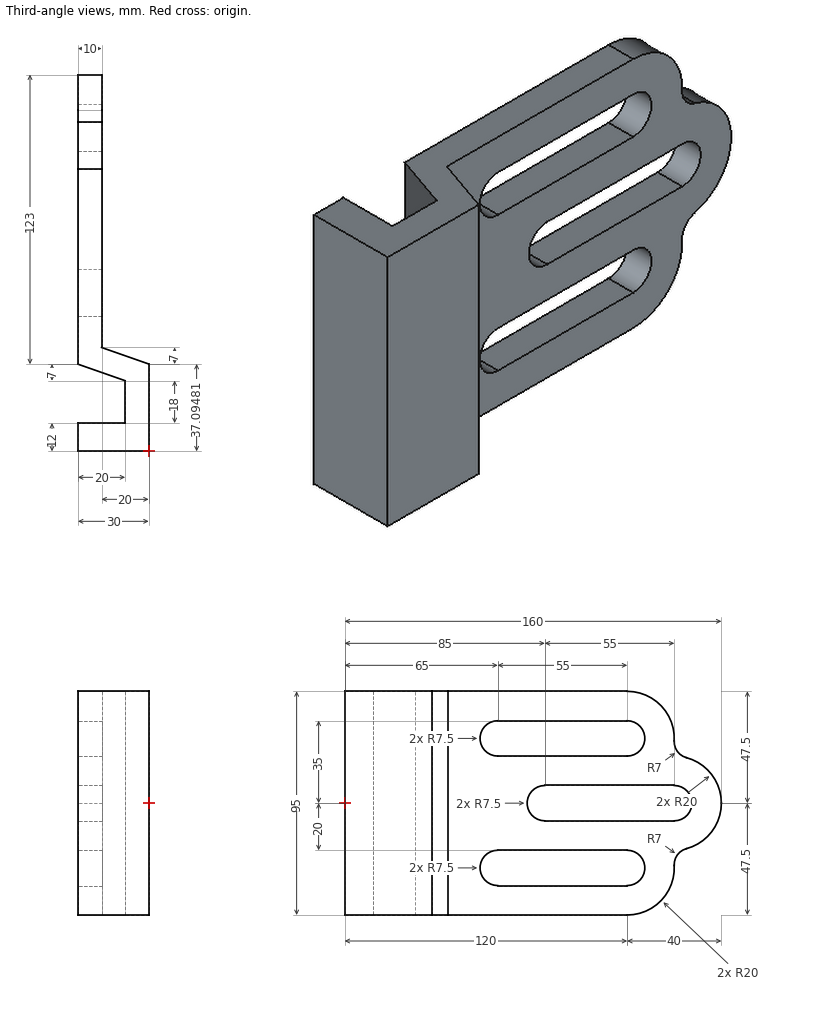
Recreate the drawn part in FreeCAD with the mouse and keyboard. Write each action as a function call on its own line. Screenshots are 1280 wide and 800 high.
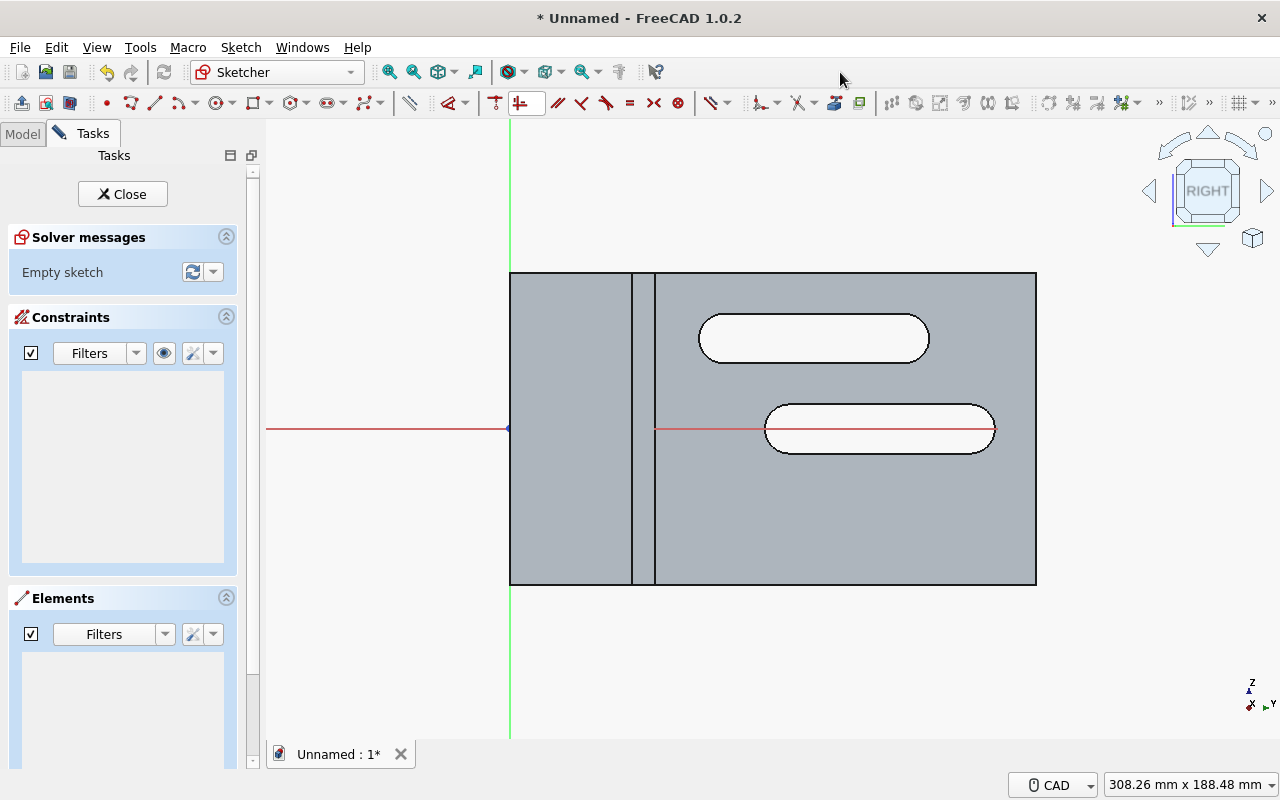
scroll(750, 604, up, 2)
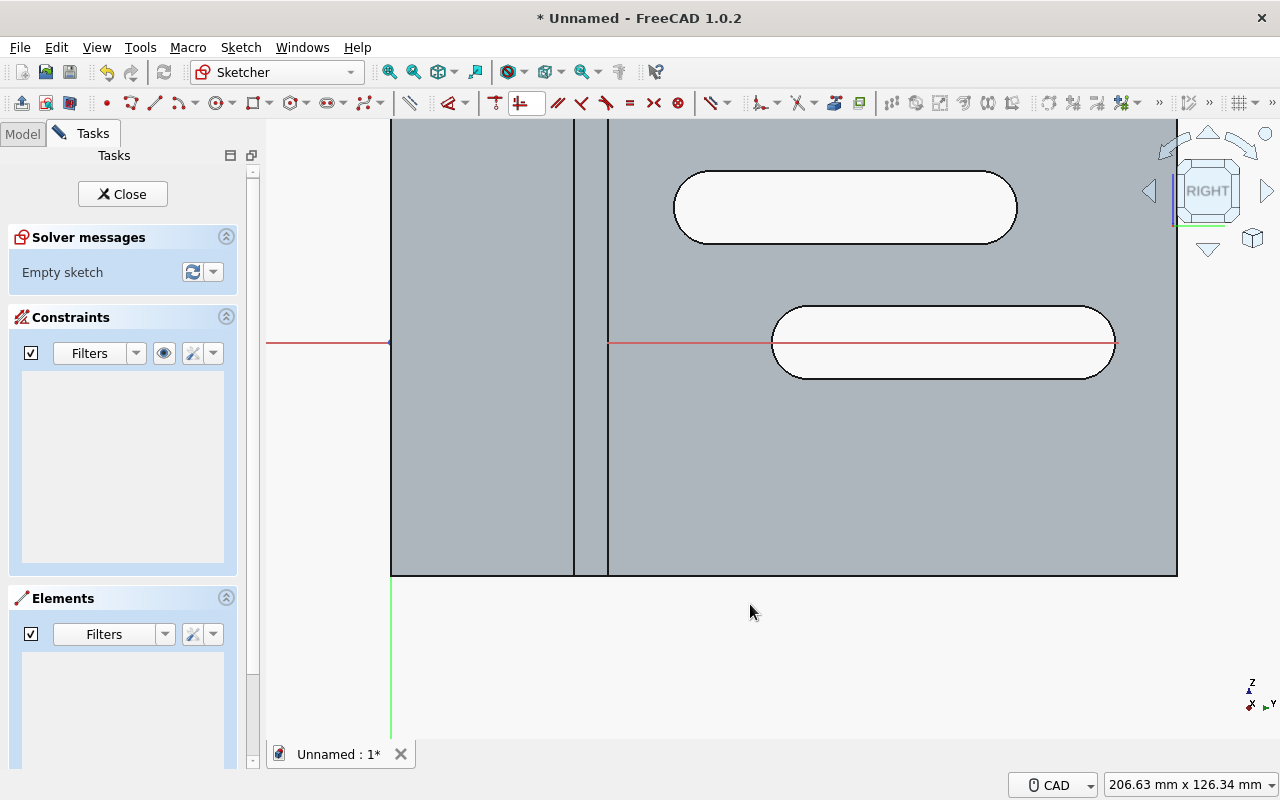
key(g)
key(s)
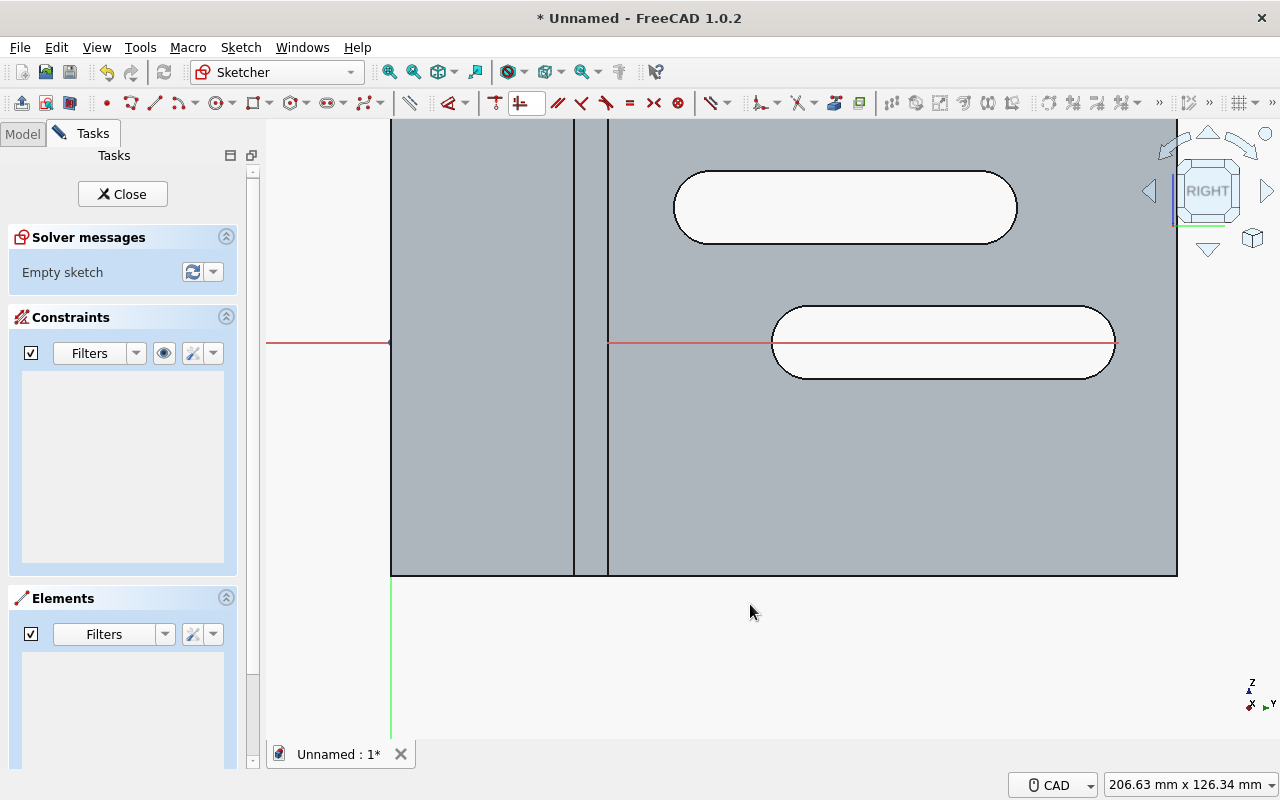
click(710, 477)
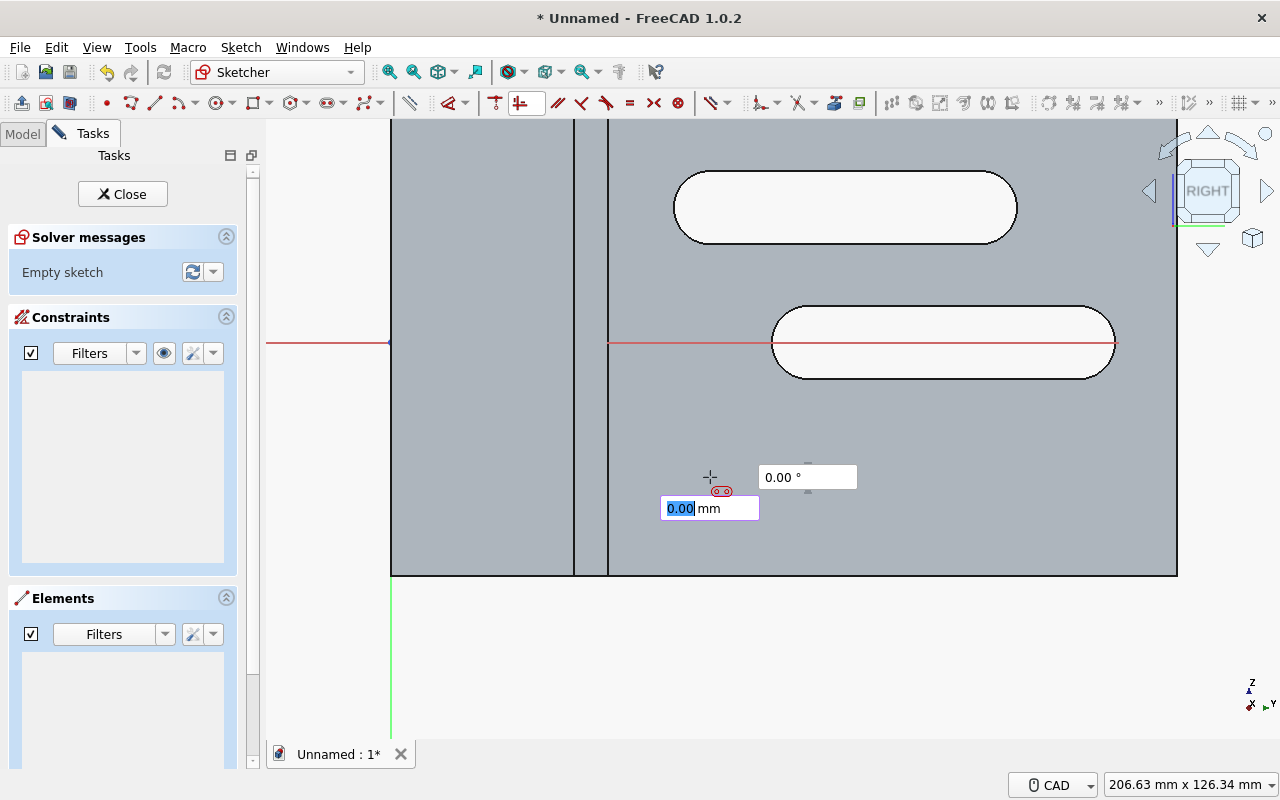
click(980, 477)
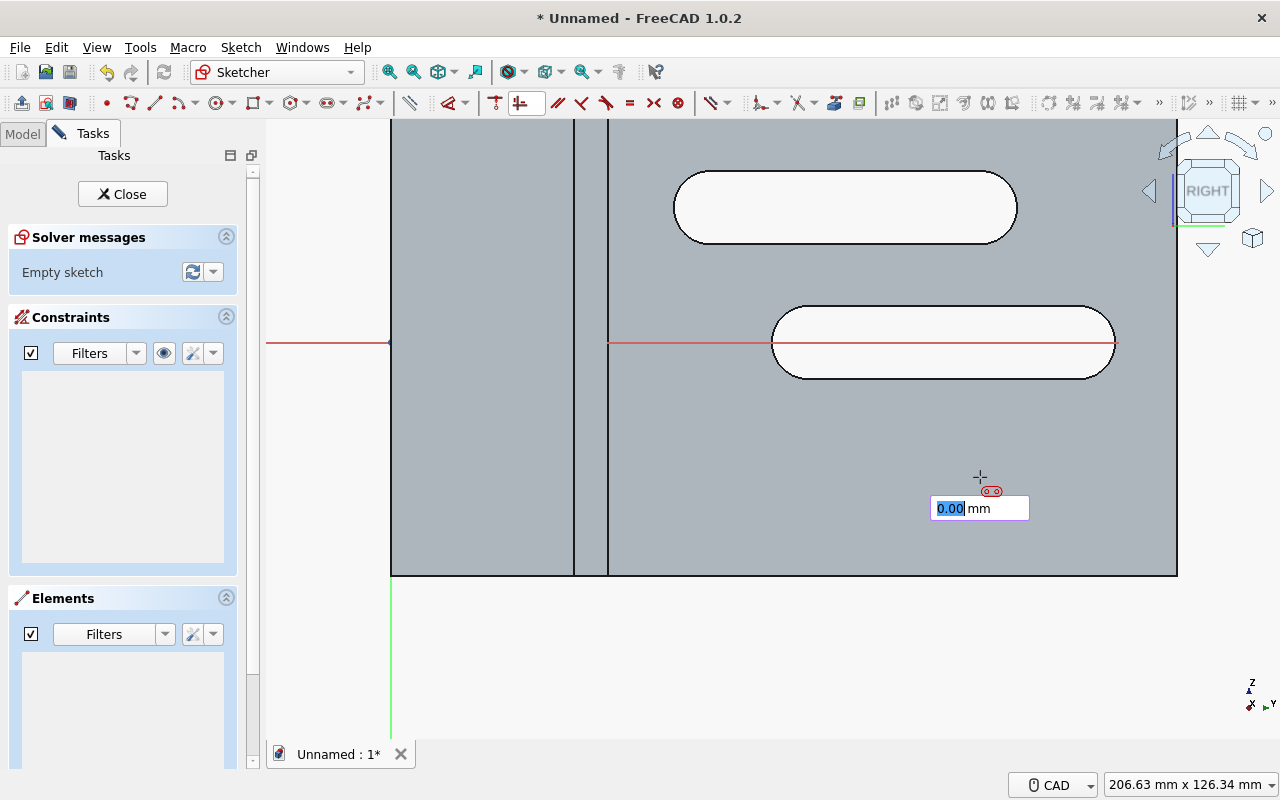
click(845, 514)
key(Escape)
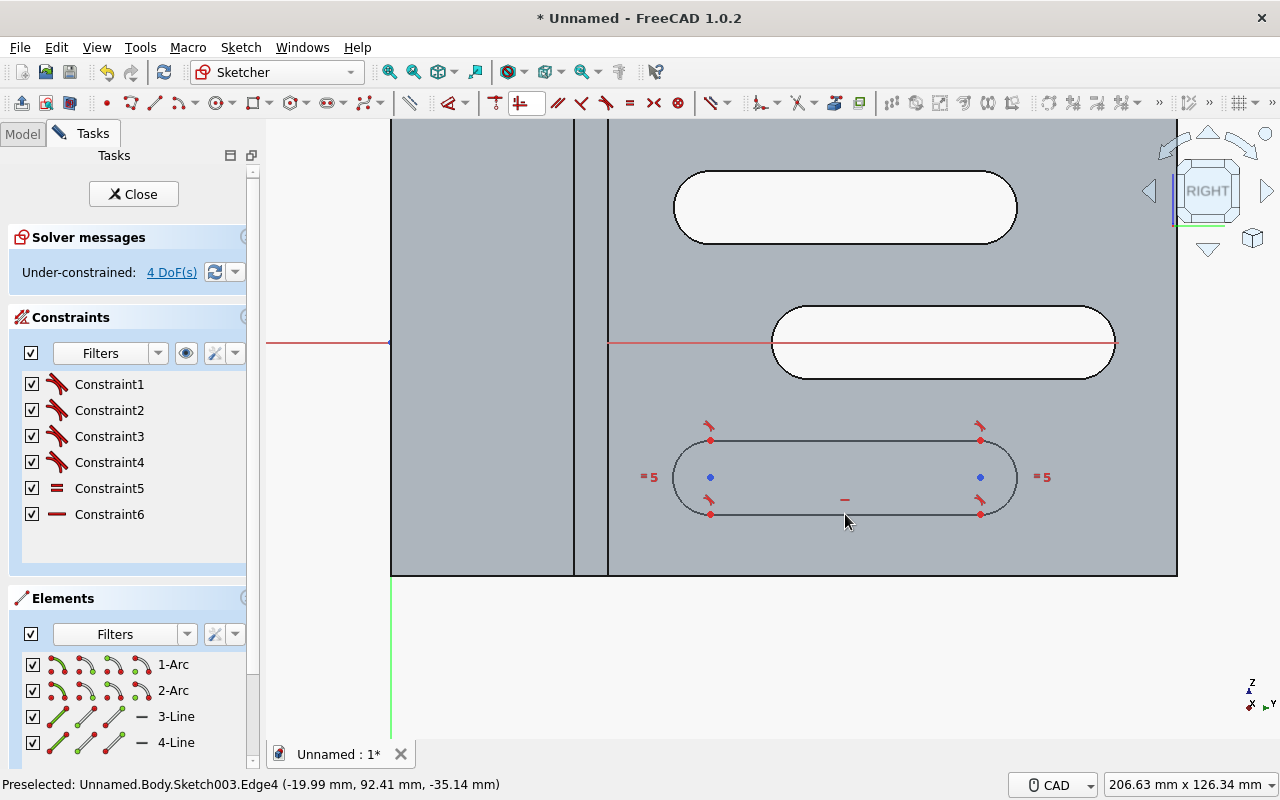
click(448, 104)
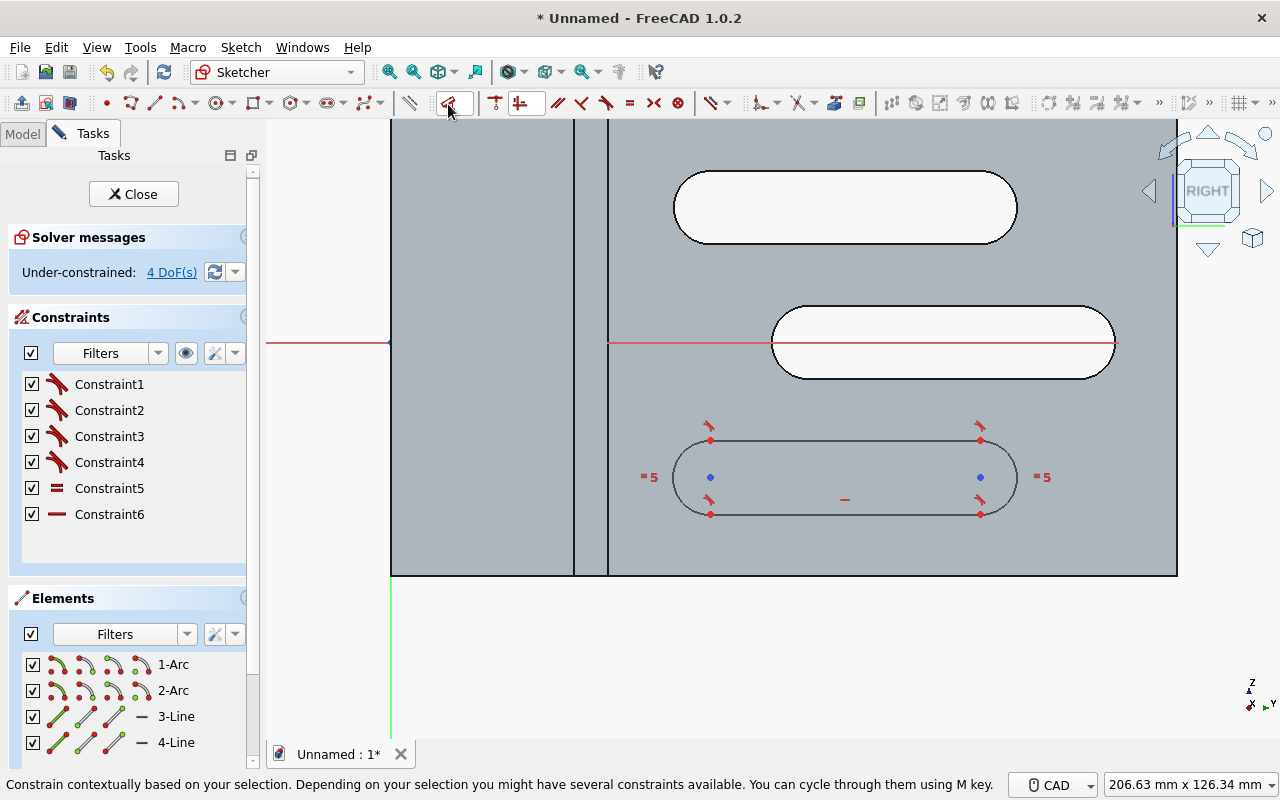
click(680, 456)
click(654, 437)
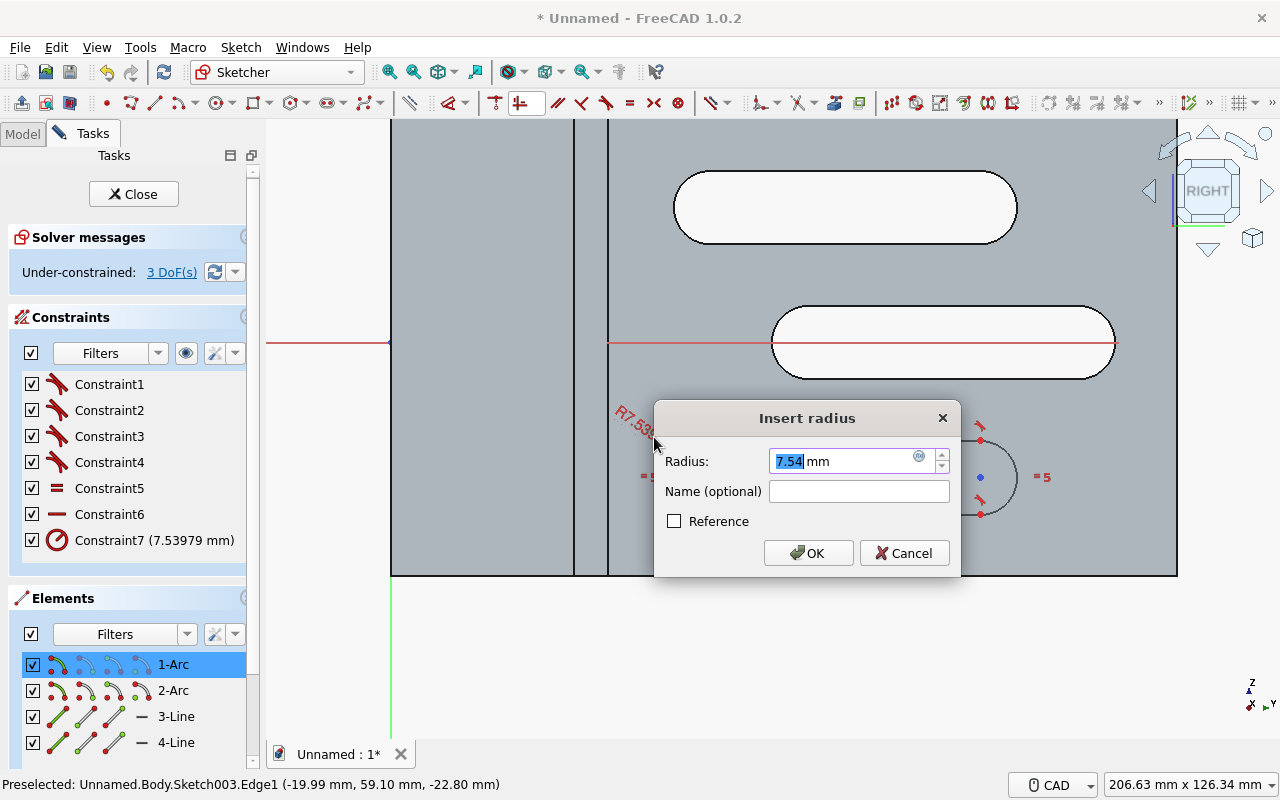
text(7.5)
key(Return)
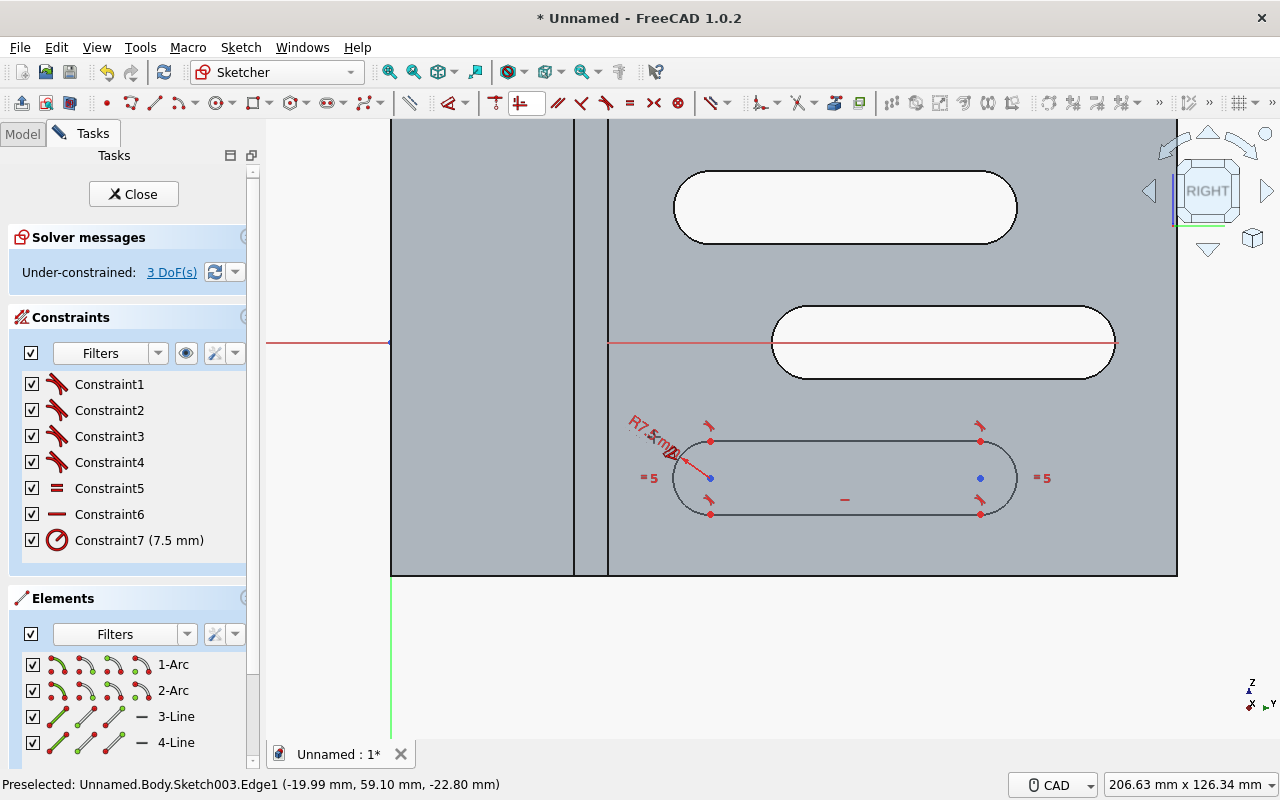
click(791, 441)
click(845, 475)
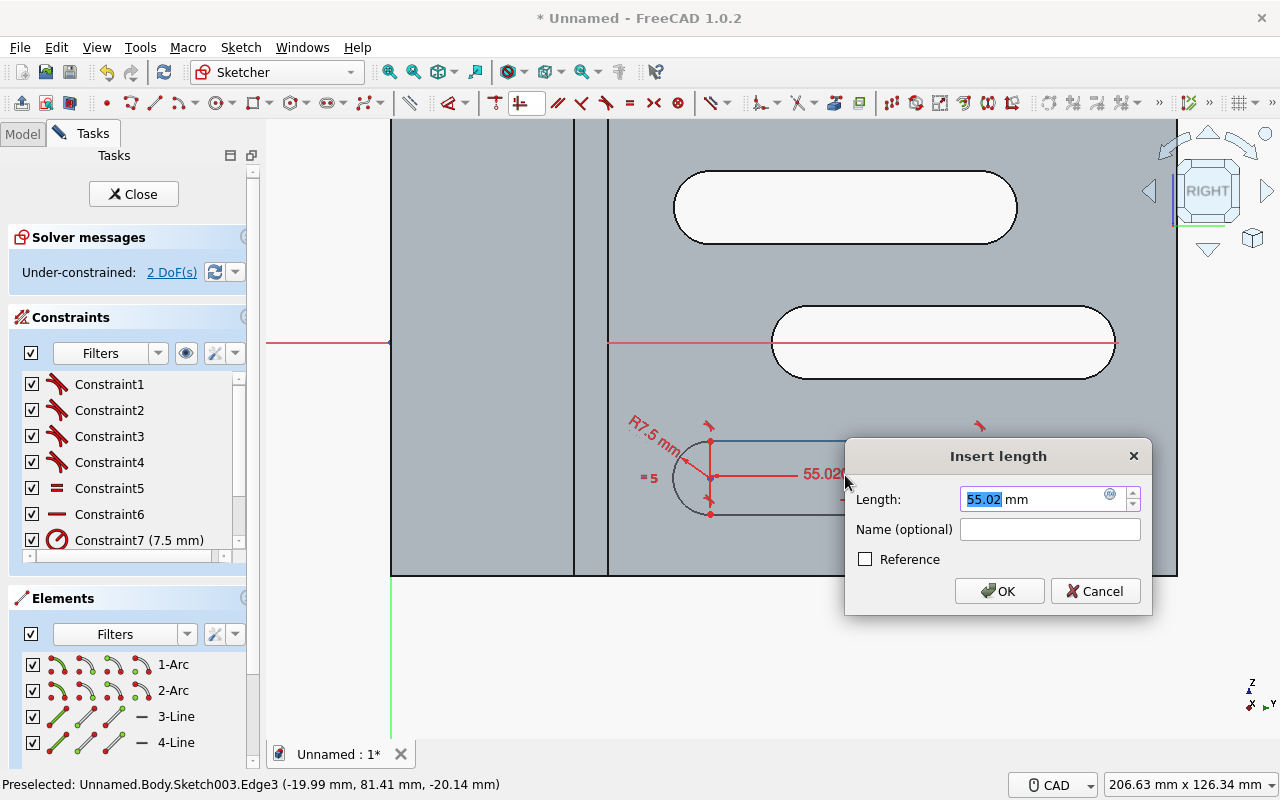
text(55)
key(Return)